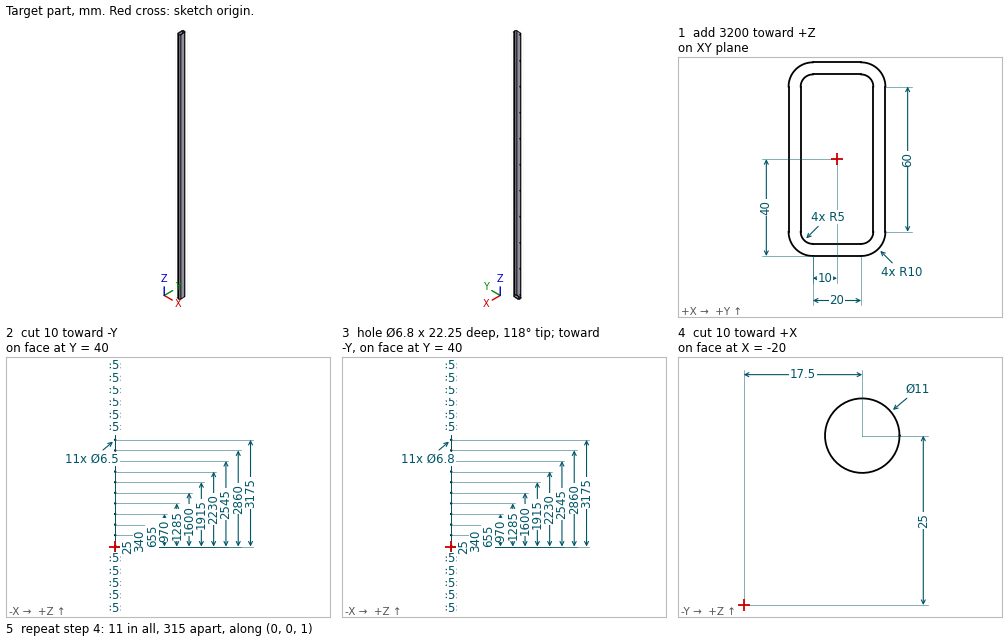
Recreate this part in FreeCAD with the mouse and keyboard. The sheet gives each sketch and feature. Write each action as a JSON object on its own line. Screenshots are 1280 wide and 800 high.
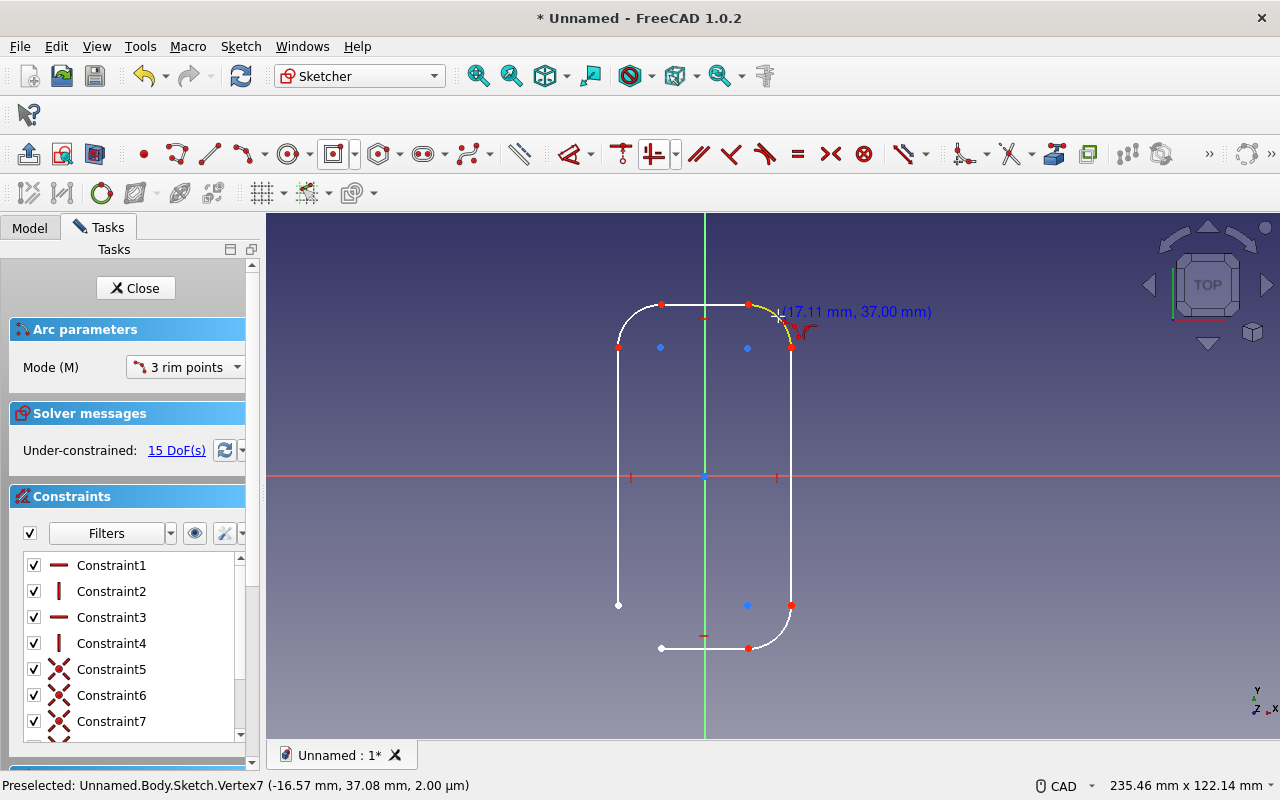
{"action": "left_click", "coordinate": [618, 606]}
{"action": "left_click", "coordinate": [661, 649]}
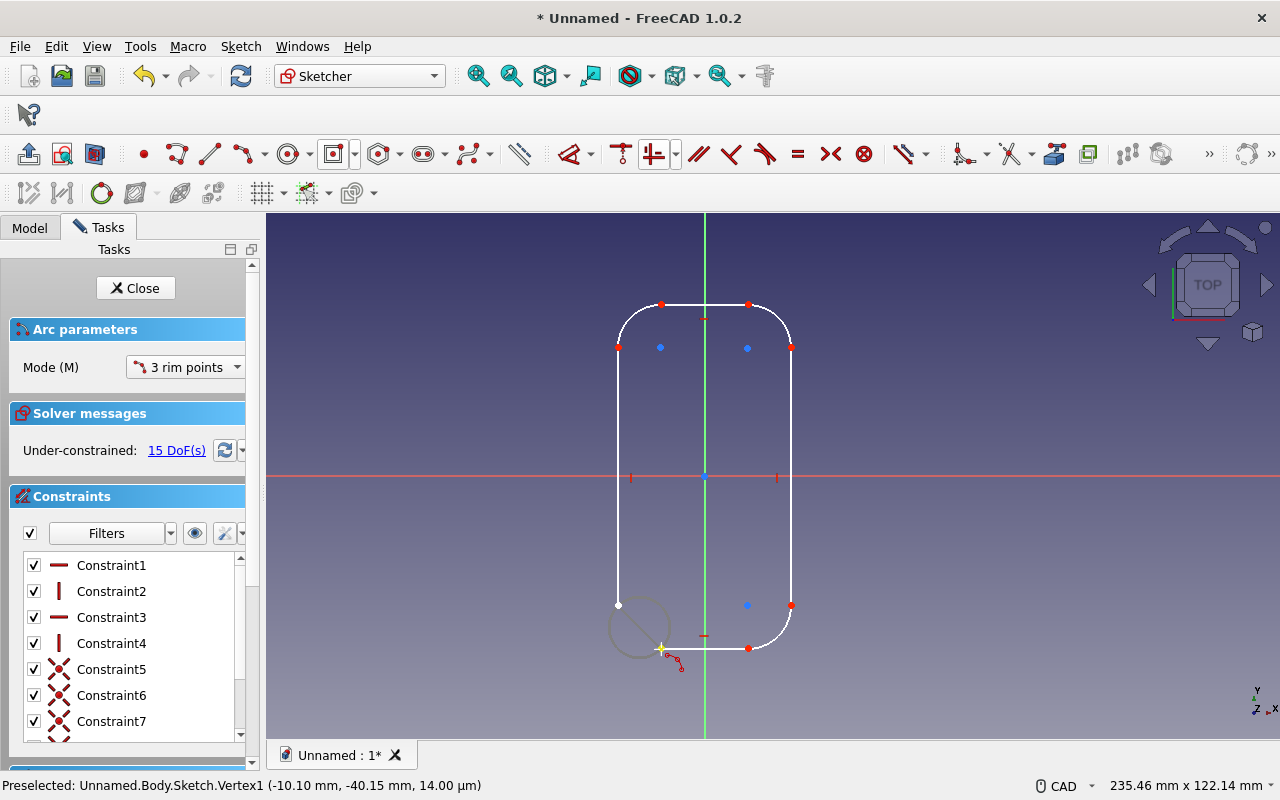
{"action": "scroll", "coordinate": [631, 636], "scroll_direction": "up", "scroll_amount": 2}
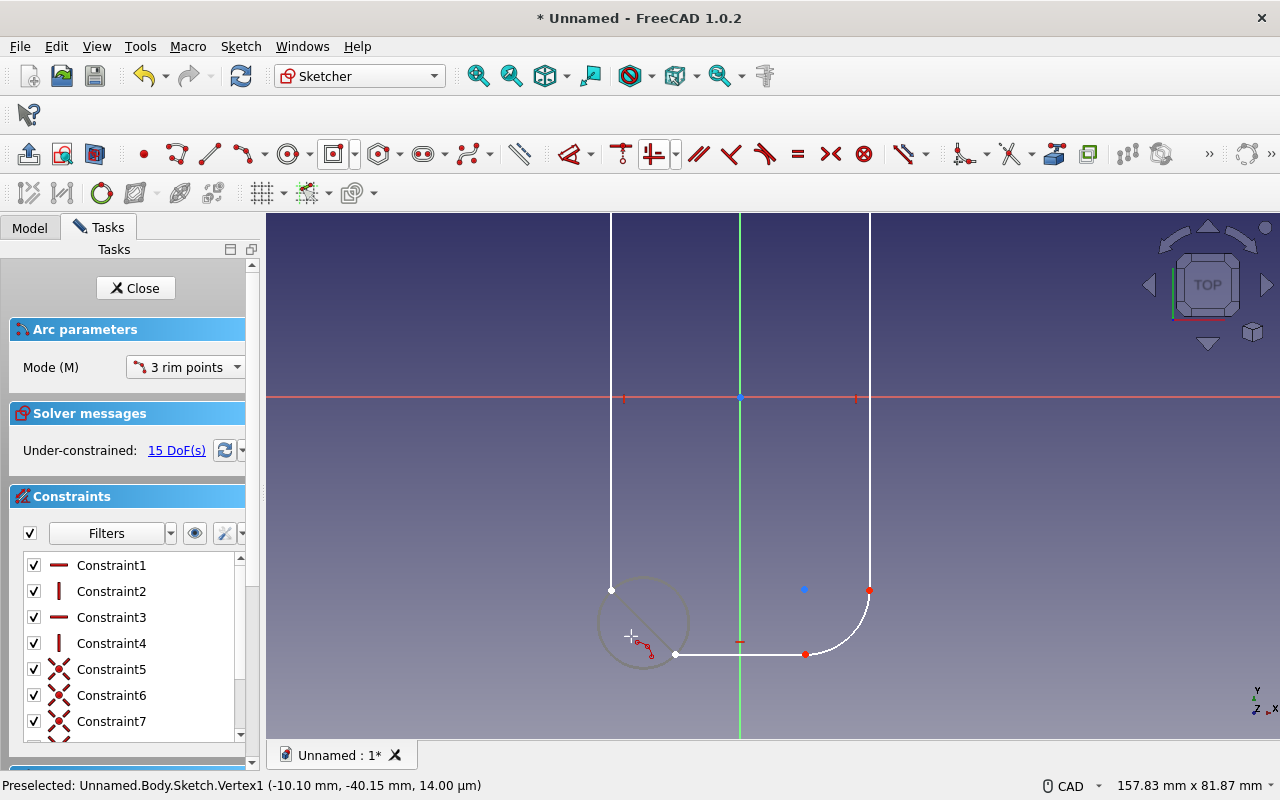
{"action": "left_click", "coordinate": [631, 635]}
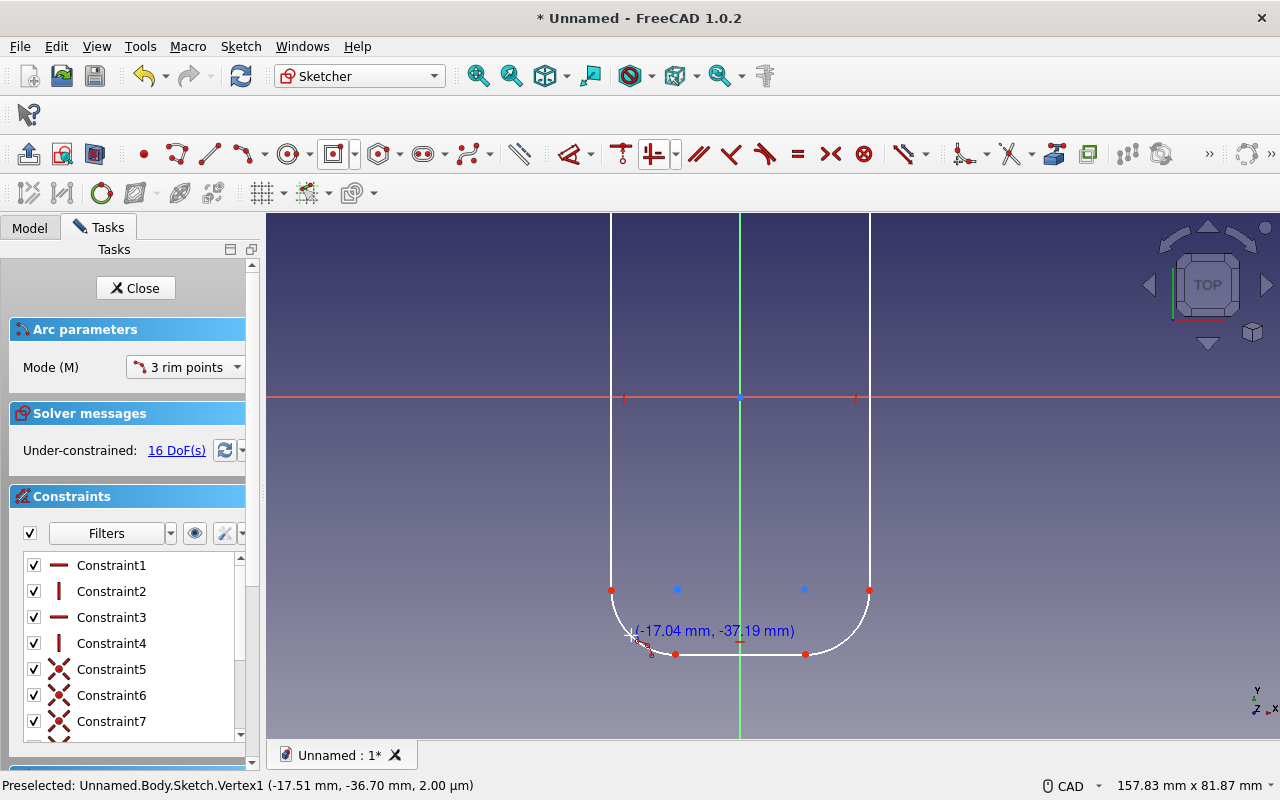
{"action": "left_click", "coordinate": [210, 154]}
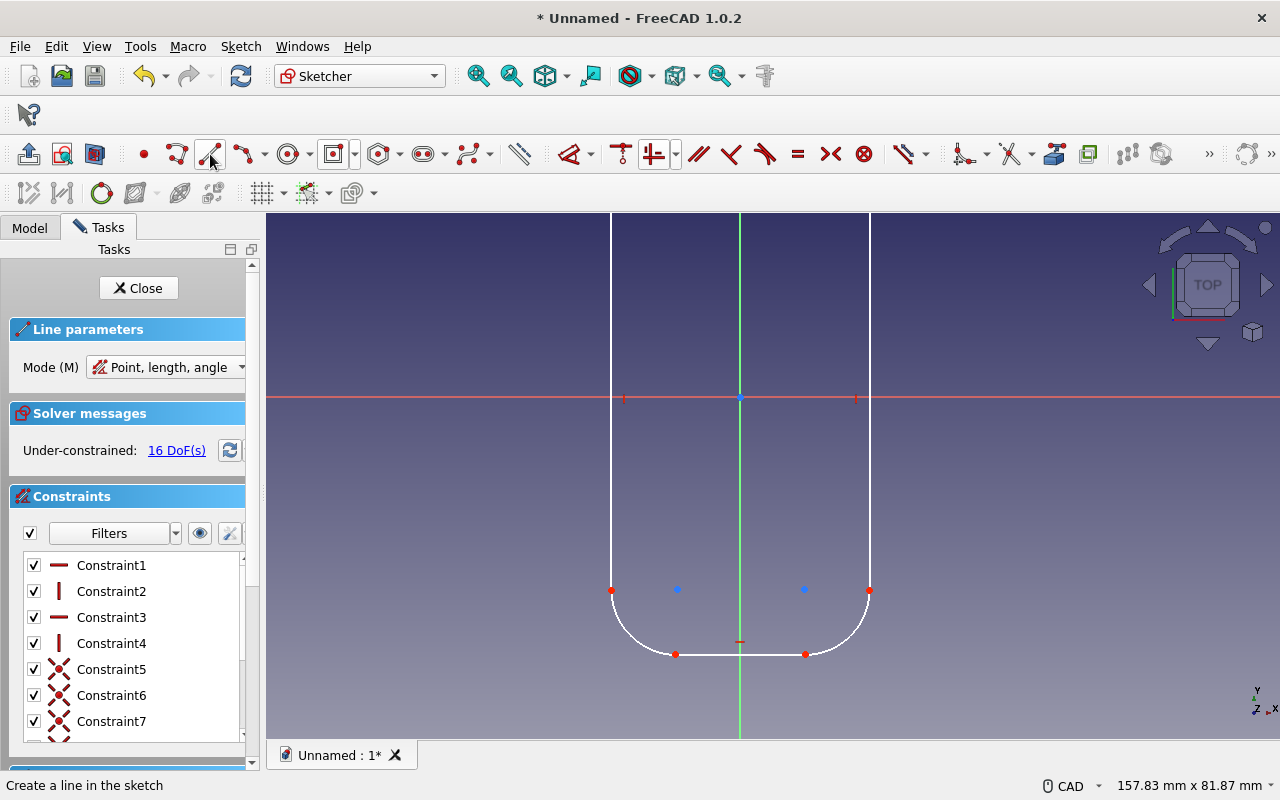
{"action": "left_click", "coordinate": [805, 622]}
{"action": "left_click", "coordinate": [676, 622]}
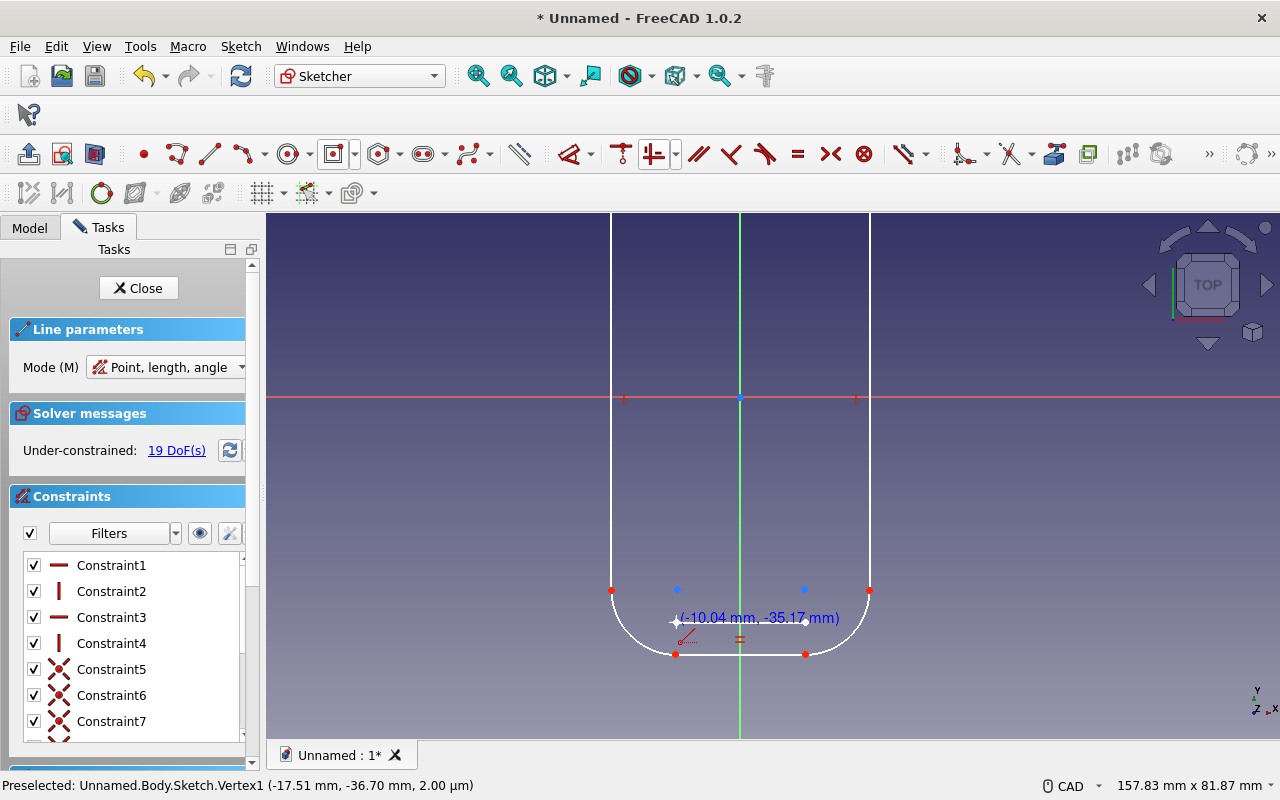
{"action": "left_click", "coordinate": [644, 590]}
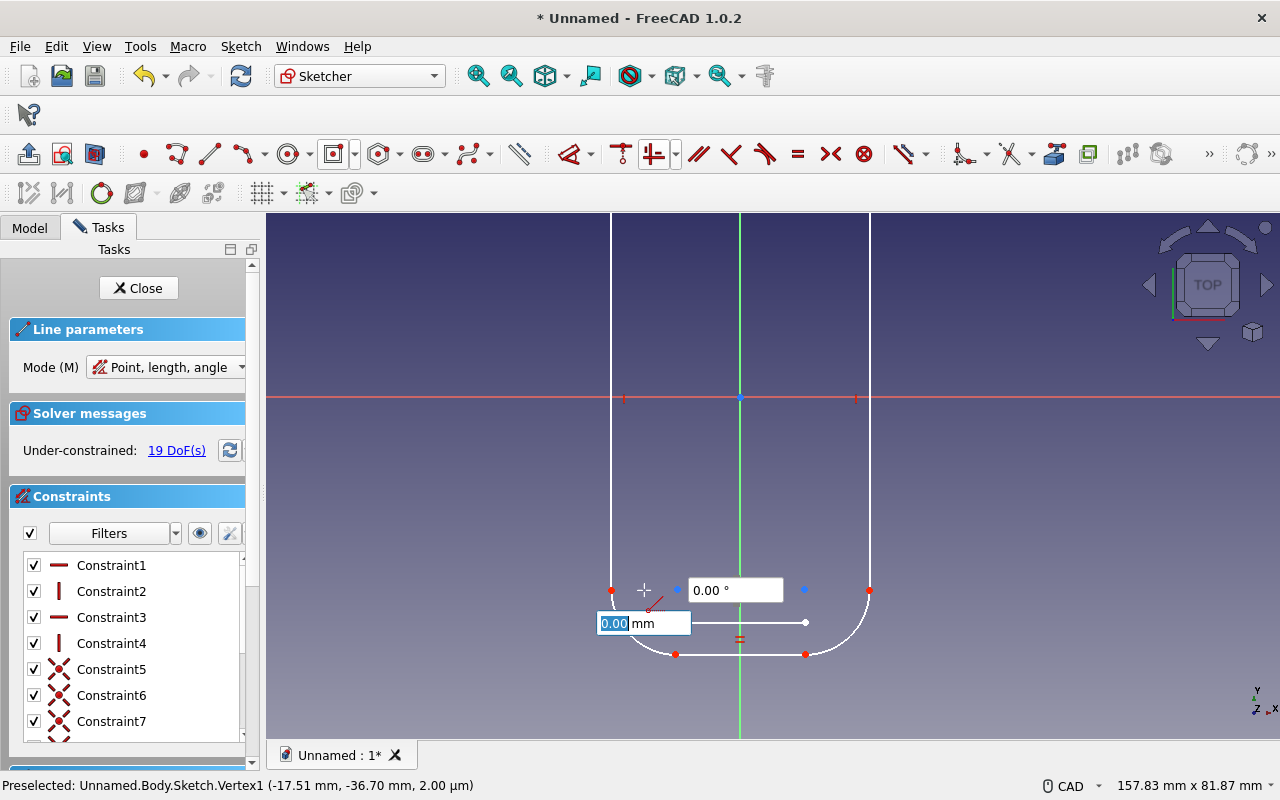
{"action": "scroll", "coordinate": [631, 637], "scroll_direction": "down", "scroll_amount": 2}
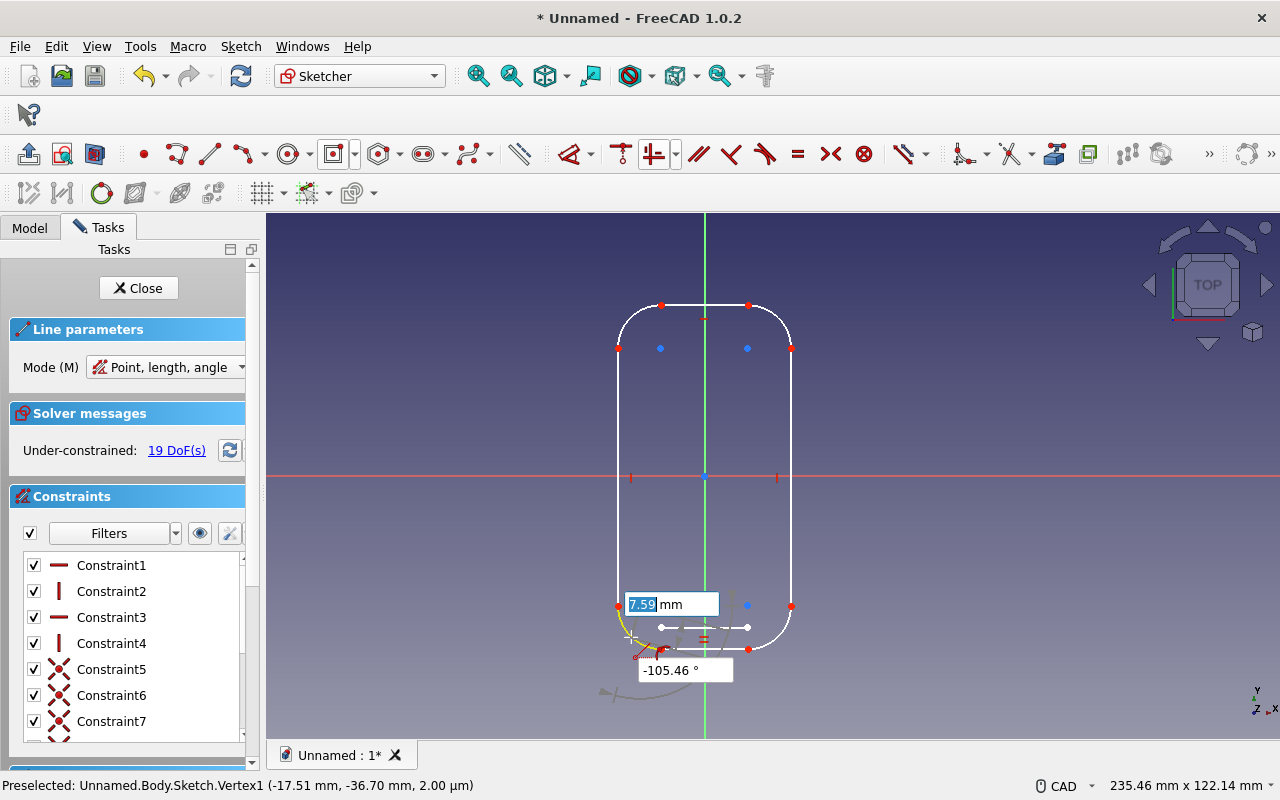
{"action": "left_click", "coordinate": [640, 347]}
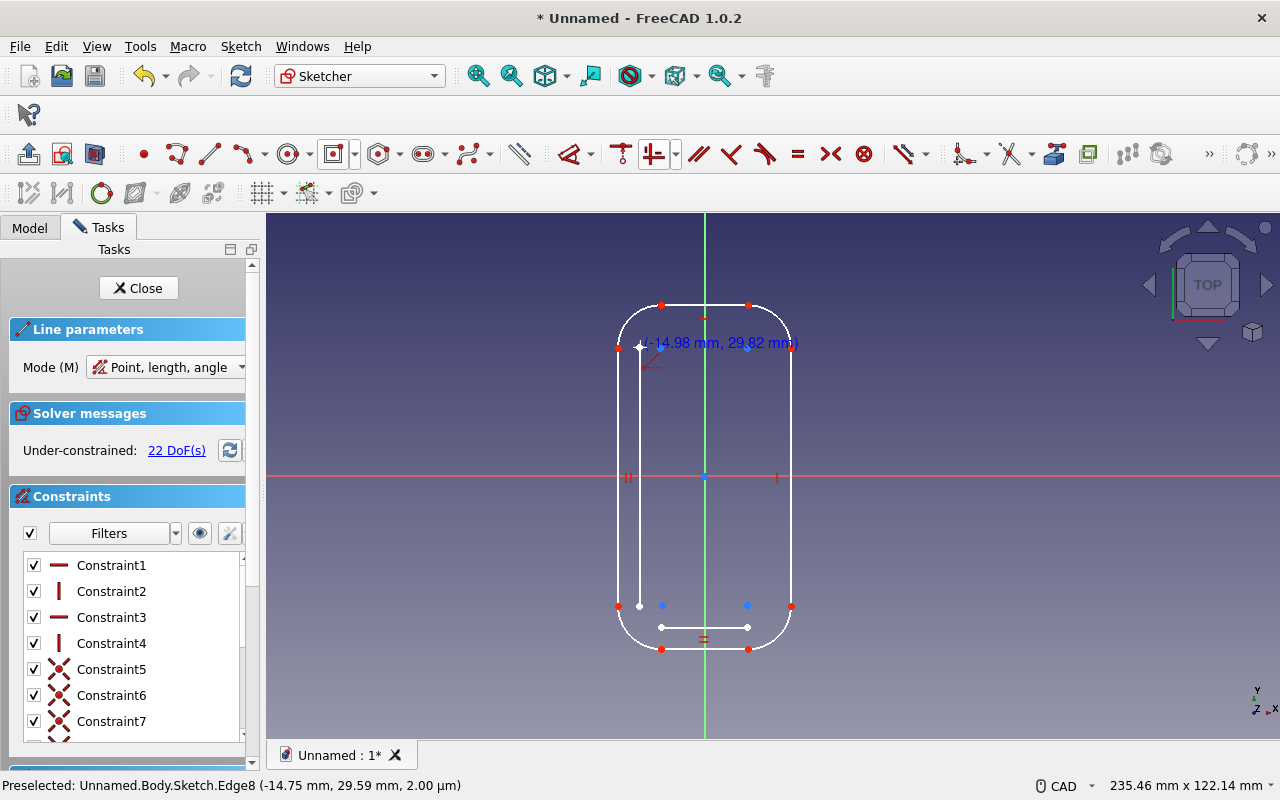
{"action": "left_click", "coordinate": [661, 326]}
{"action": "left_click", "coordinate": [748, 326]}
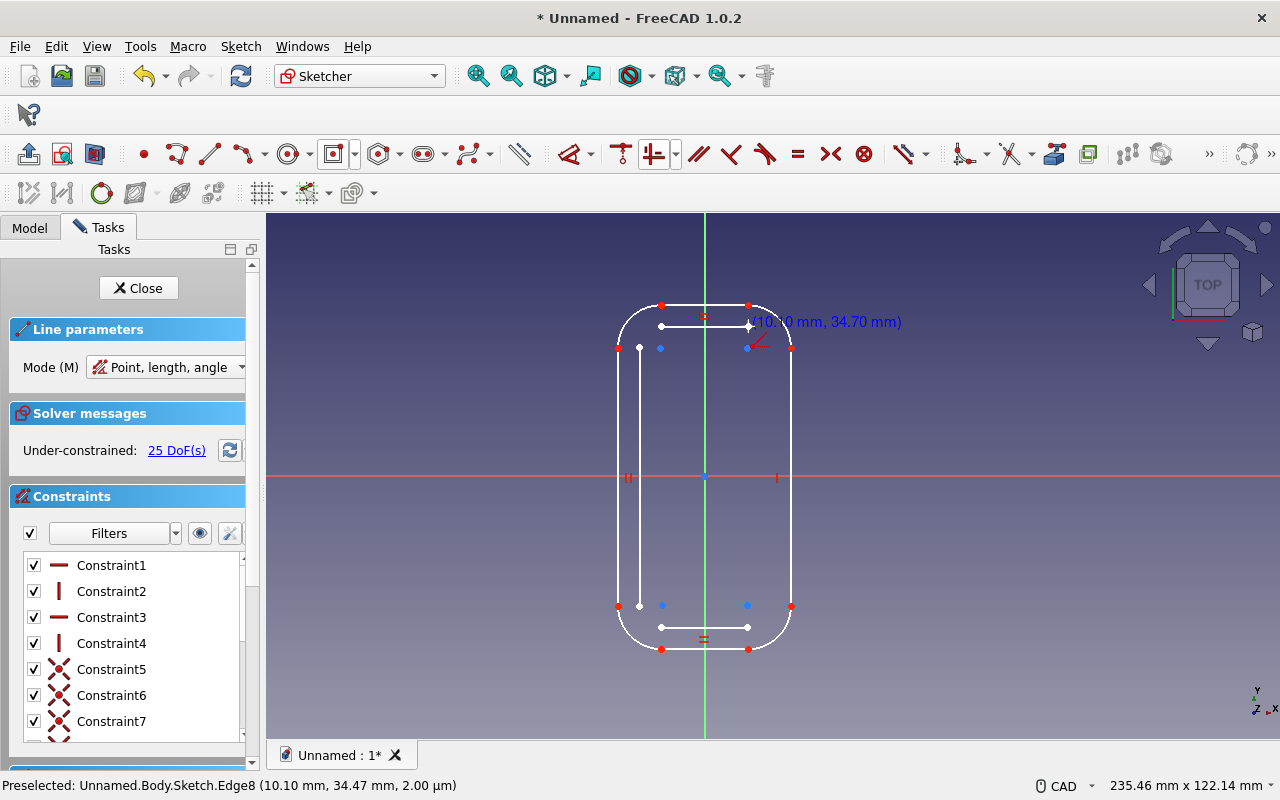
{"action": "left_click", "coordinate": [769, 347]}
{"action": "left_click", "coordinate": [769, 606]}